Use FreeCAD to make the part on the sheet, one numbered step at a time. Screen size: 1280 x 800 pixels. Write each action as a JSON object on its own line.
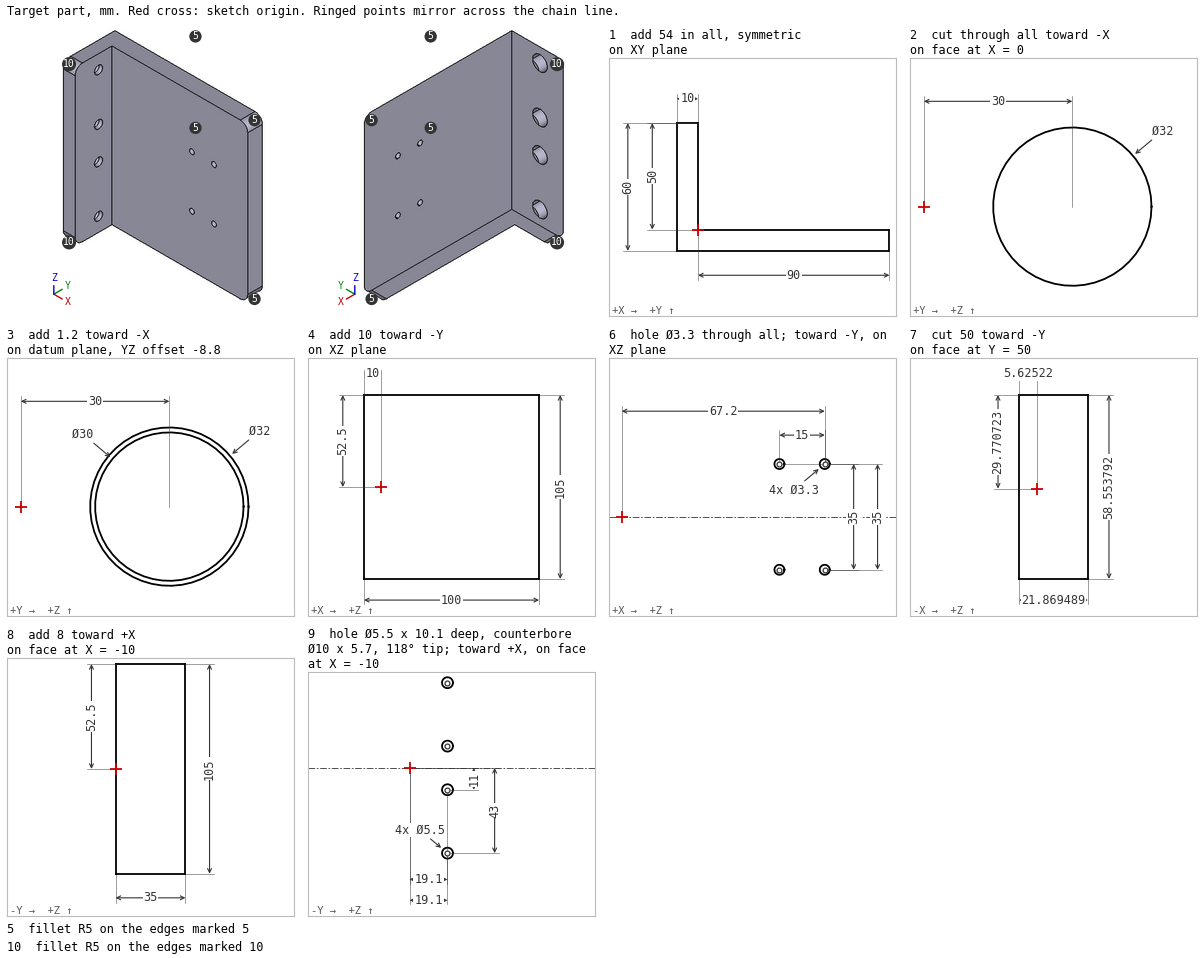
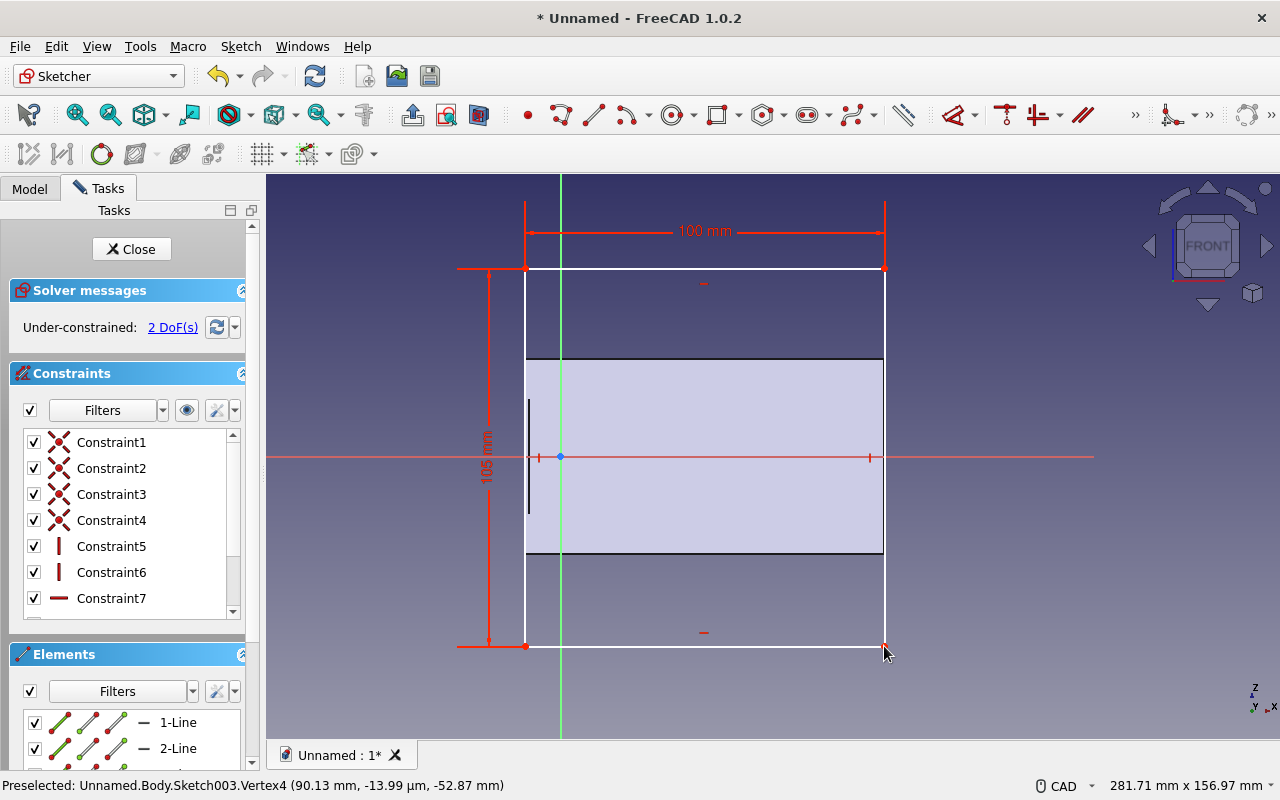
{"action": "left_click", "coordinate": [952, 116]}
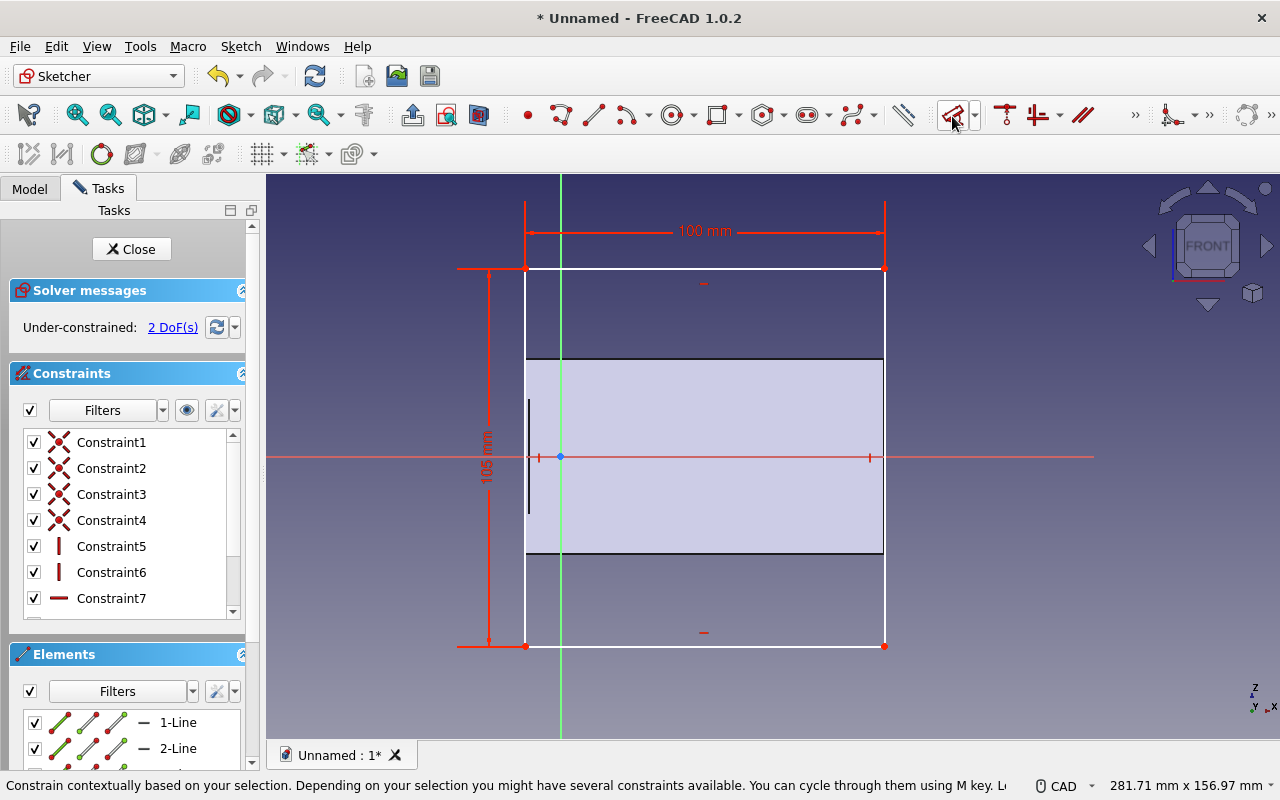
{"action": "left_click", "coordinate": [525, 269]}
{"action": "left_click", "coordinate": [543, 235]}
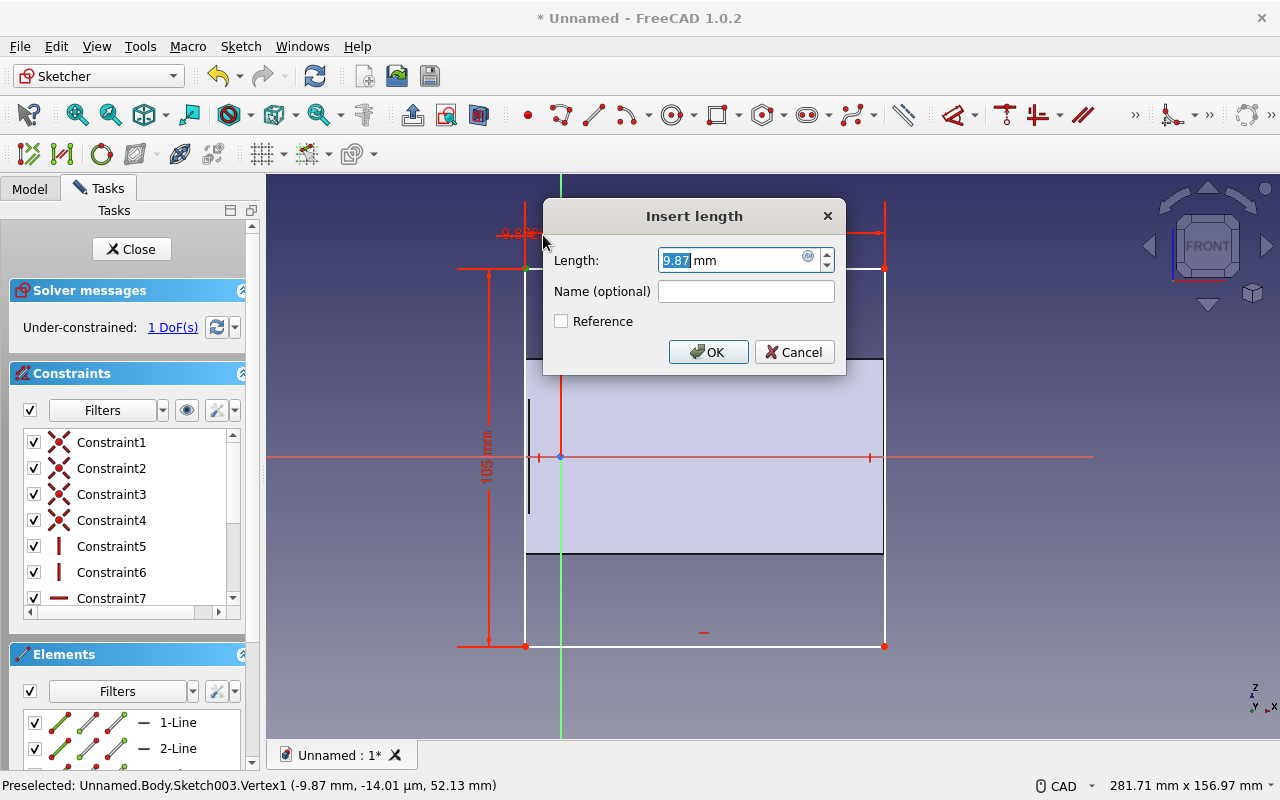
{"action": "type", "text": "10"}
{"action": "key", "text": "Return"}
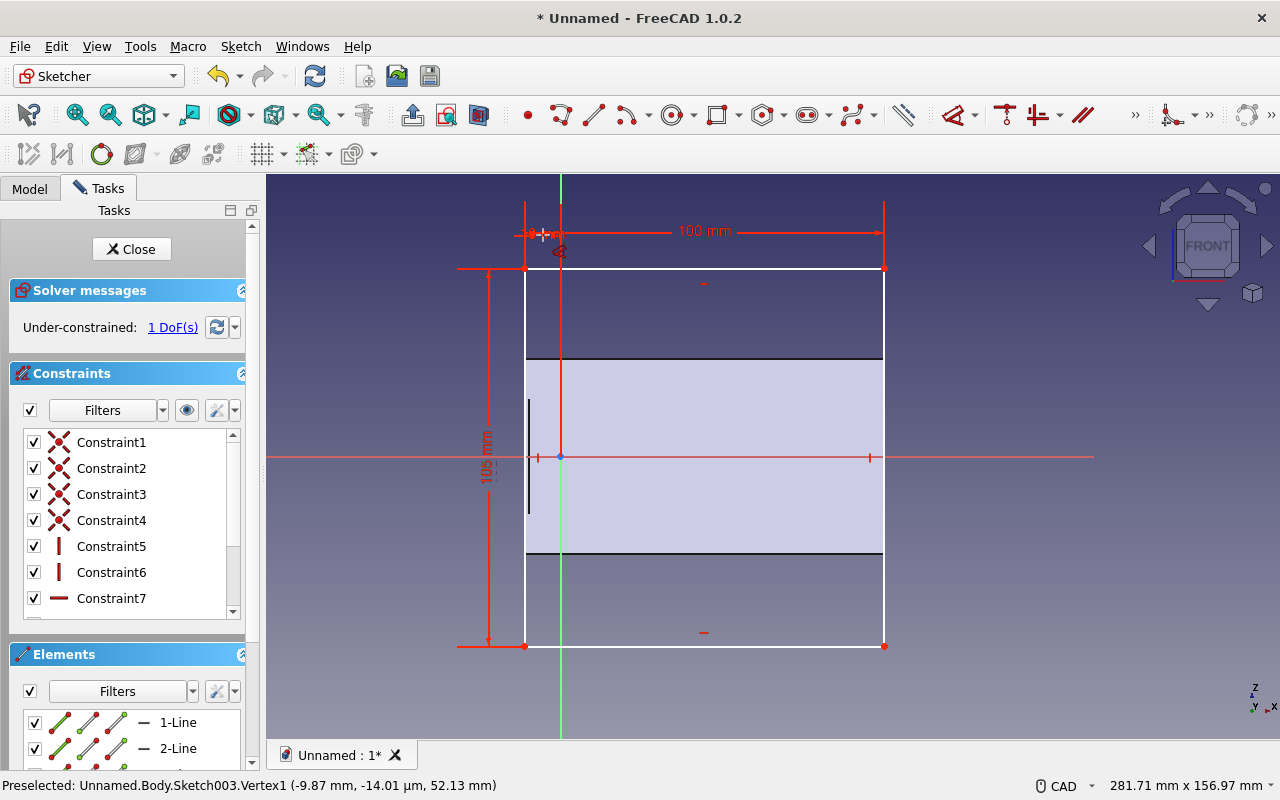
{"action": "left_click", "coordinate": [525, 269]}
{"action": "left_click", "coordinate": [491, 363]}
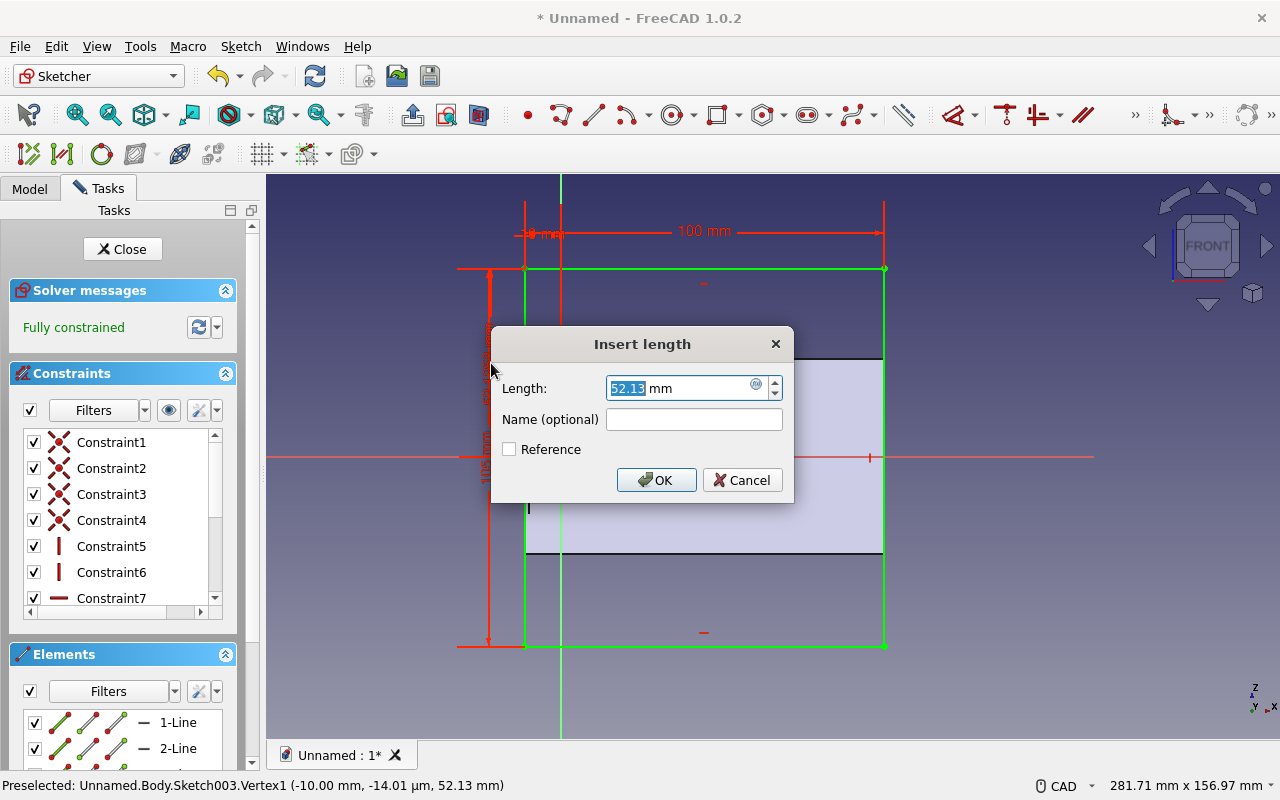
{"action": "type", "text": "52.5"}
{"action": "key", "text": "Return"}
{"action": "key", "text": "Escape"}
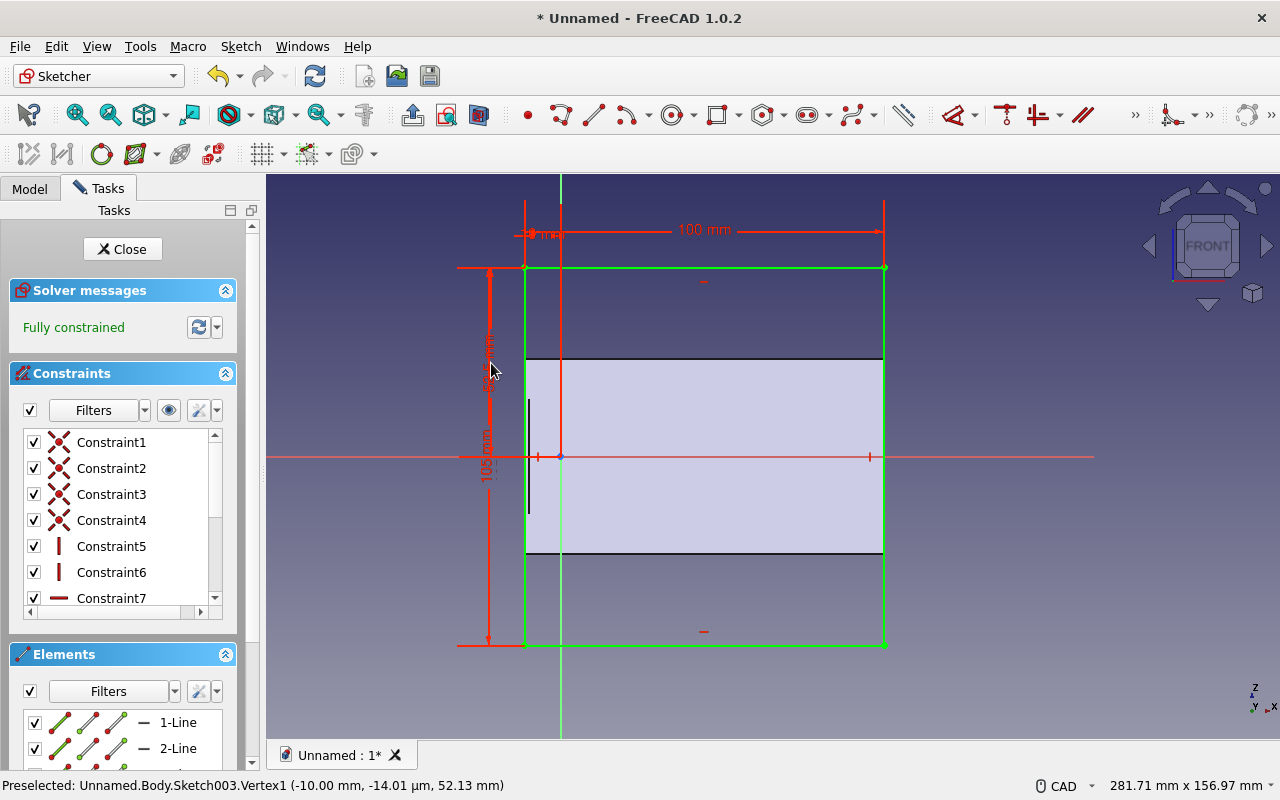
{"action": "left_click", "coordinate": [123, 249]}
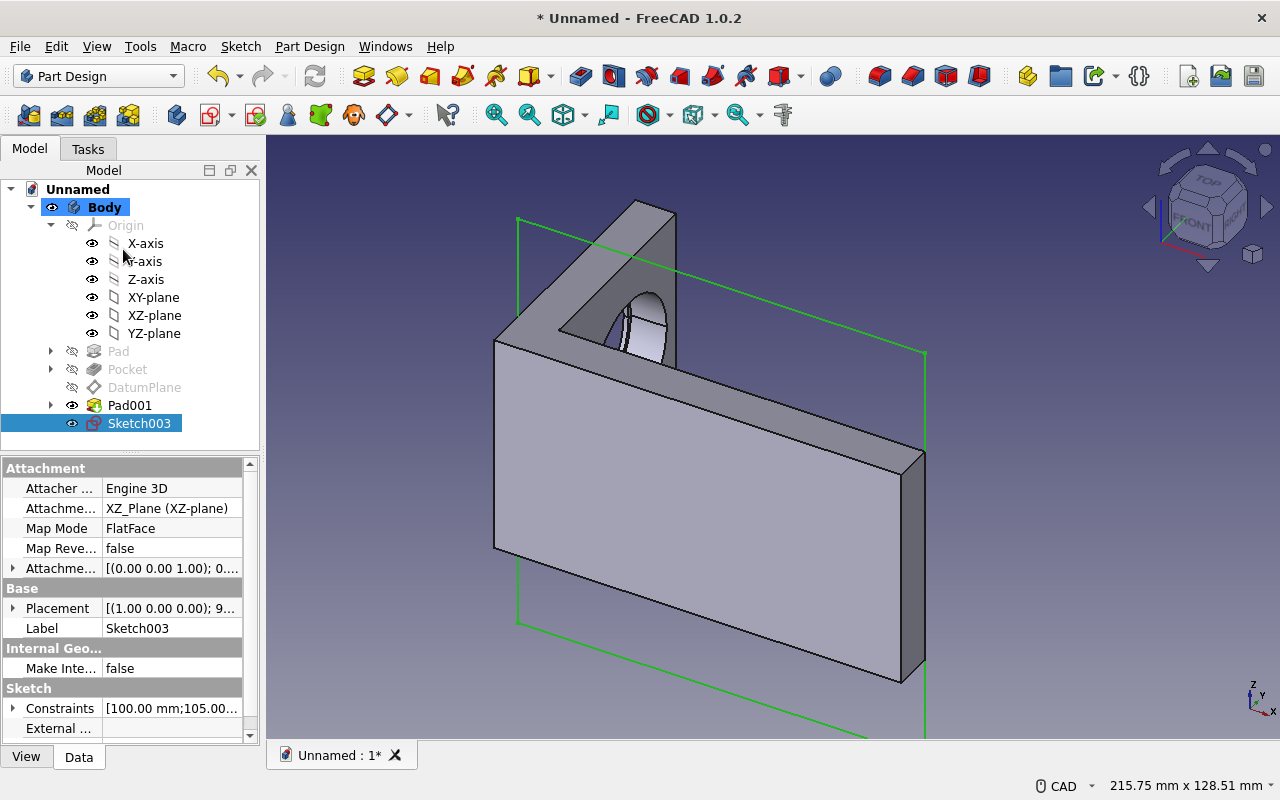
{"action": "left_click", "coordinate": [364, 76]}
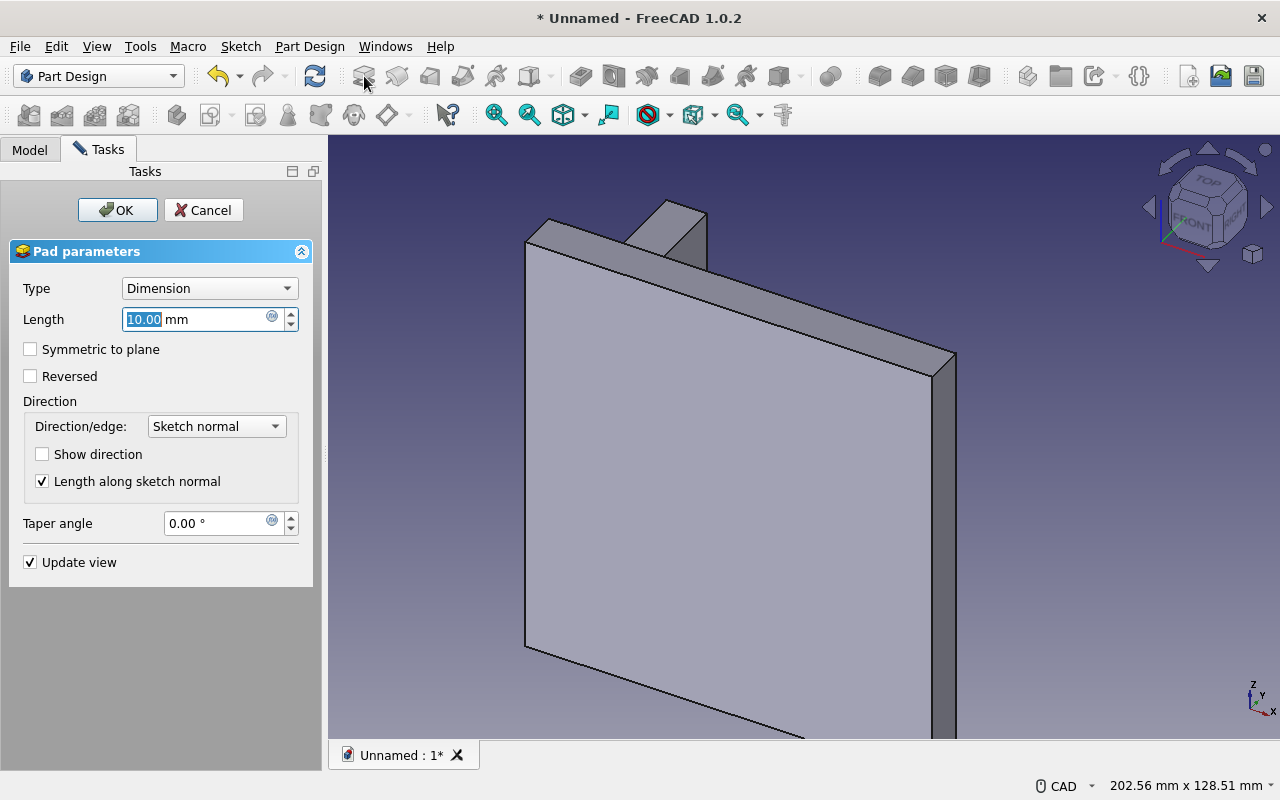
{"action": "type", "text": "10"}
{"action": "key", "text": "Tab"}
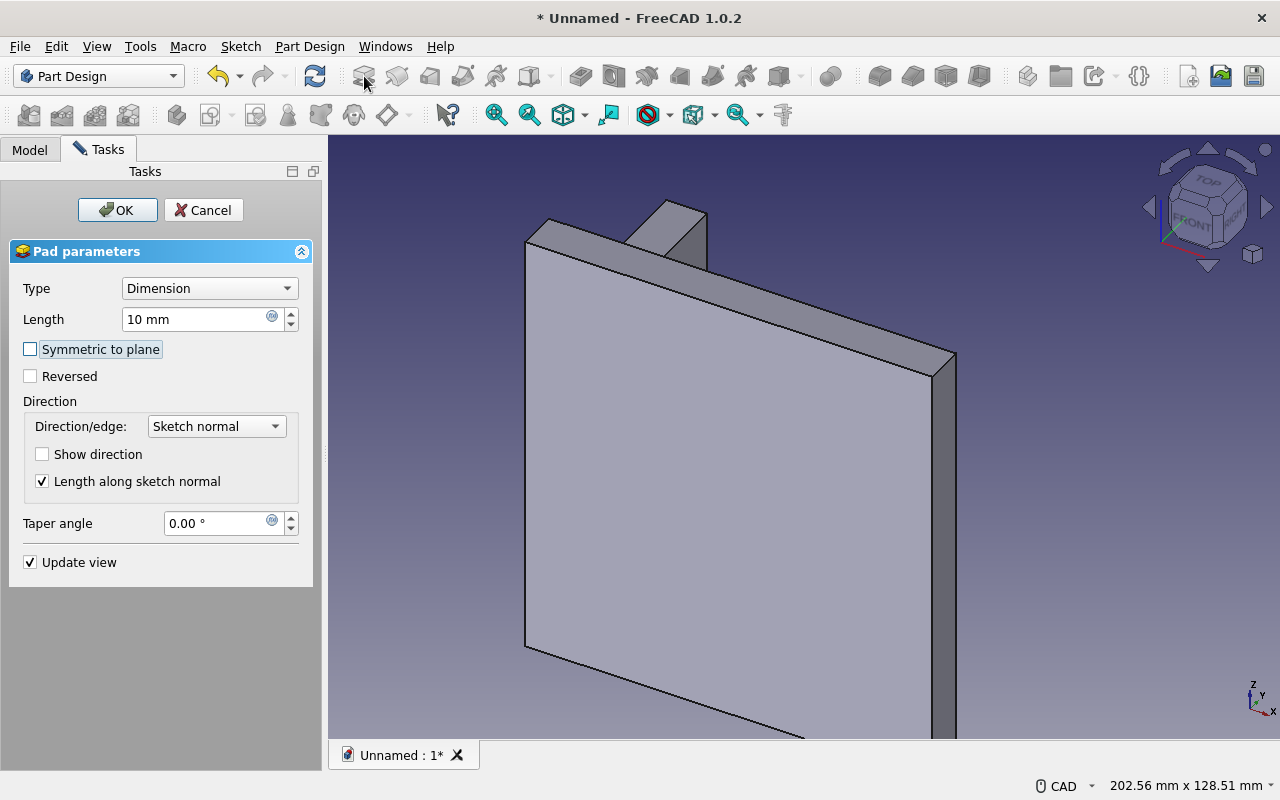
{"action": "left_click", "coordinate": [118, 210]}